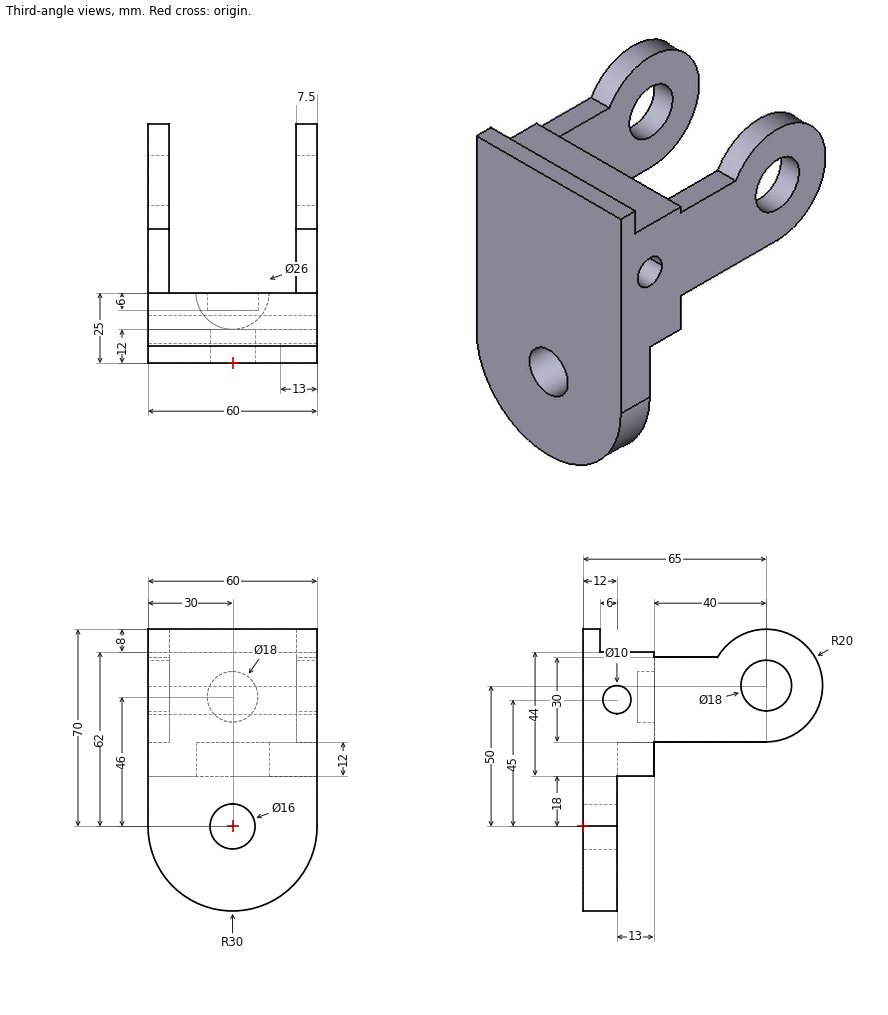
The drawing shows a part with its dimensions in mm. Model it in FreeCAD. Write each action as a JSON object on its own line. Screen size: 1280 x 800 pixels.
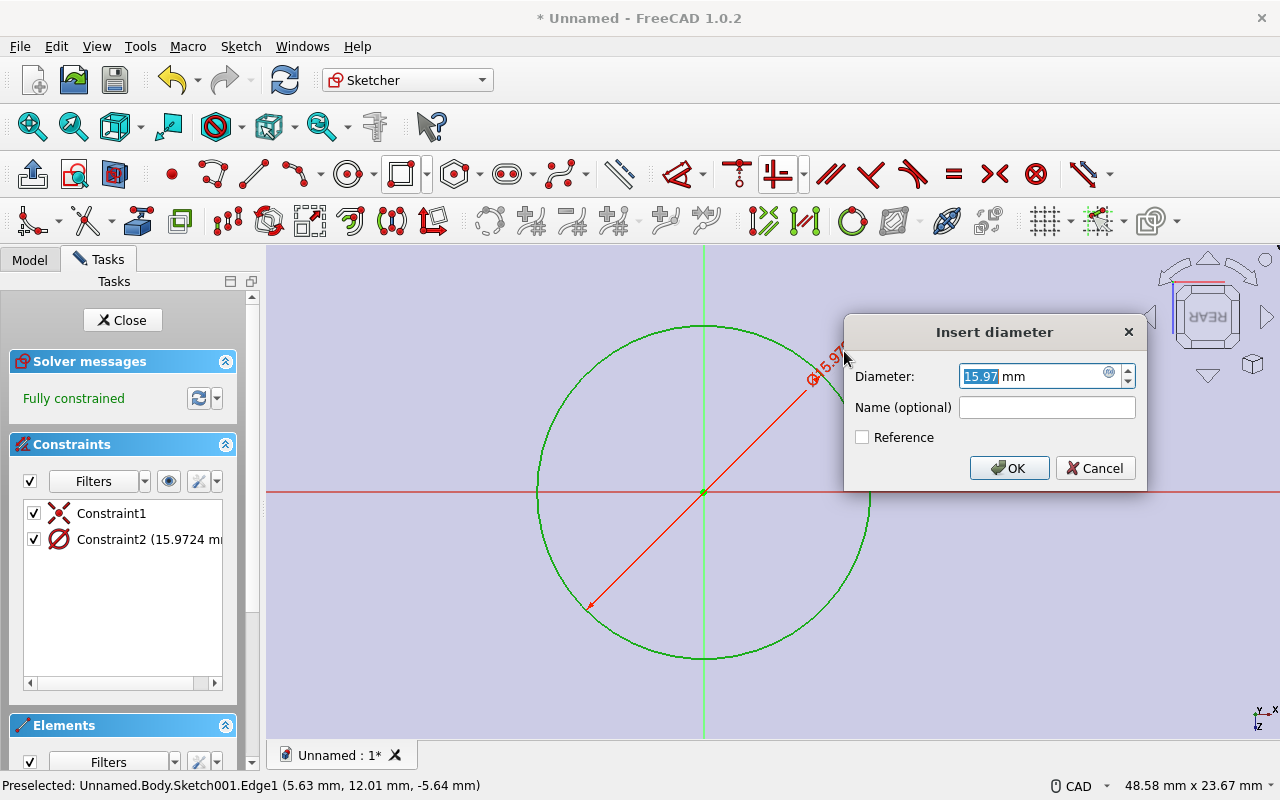
{"action": "type", "text": "16"}
{"action": "key", "text": "Return"}
{"action": "key", "text": "Escape"}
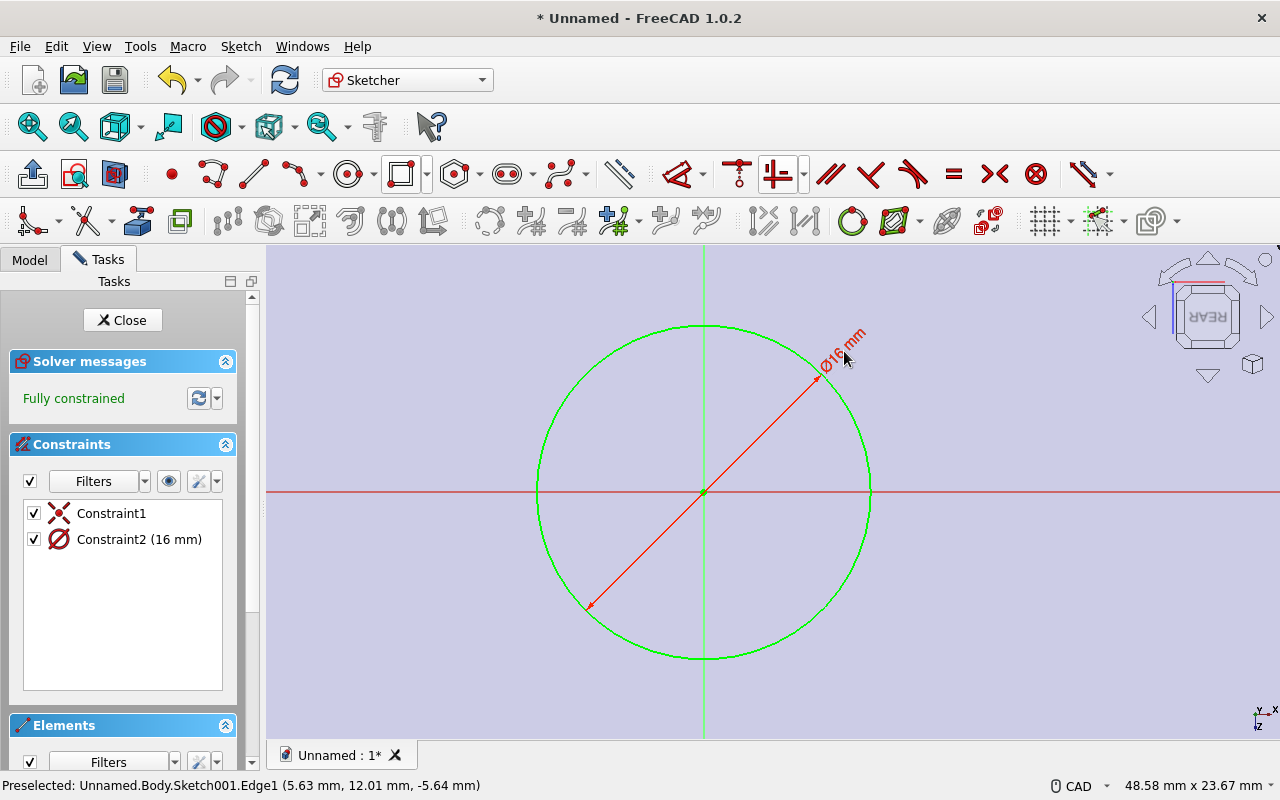
{"action": "left_click", "coordinate": [123, 320]}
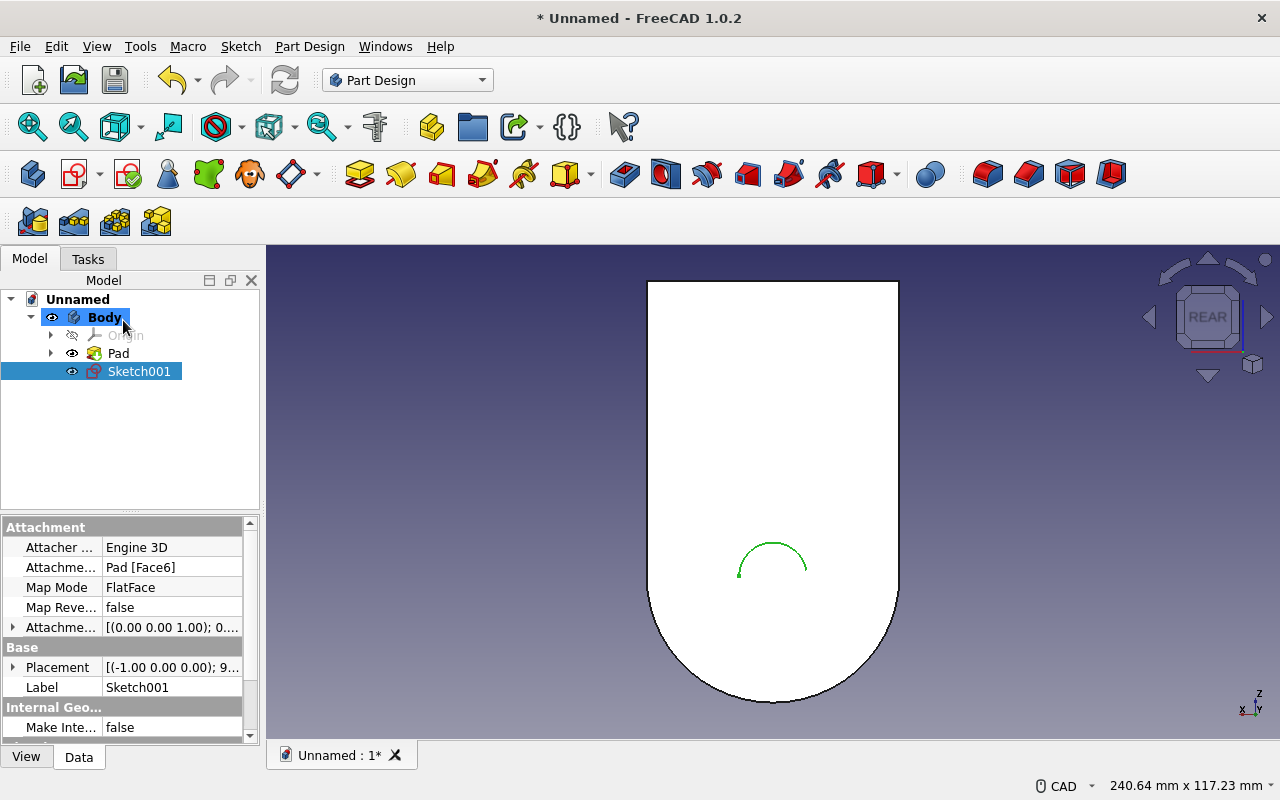
{"action": "left_click", "coordinate": [625, 174]}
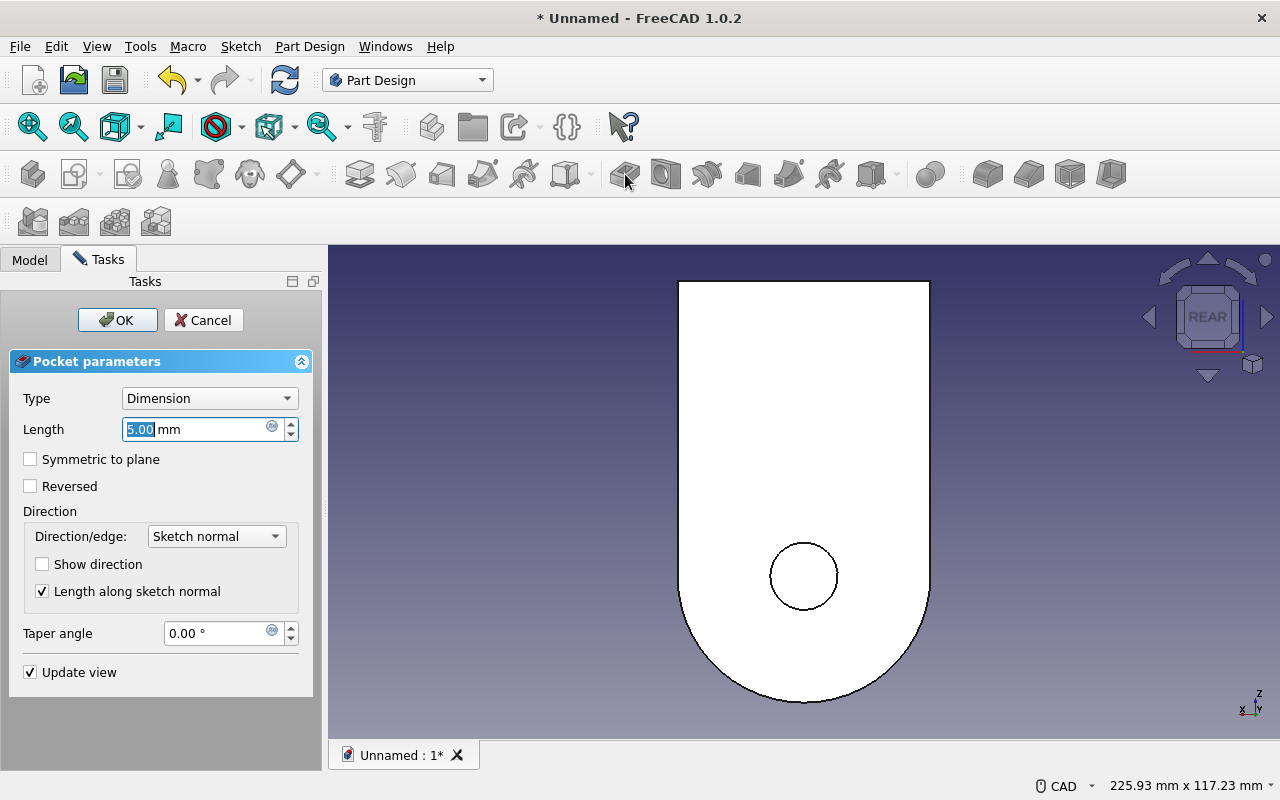
{"action": "type", "text": "12"}
{"action": "key", "text": "Tab"}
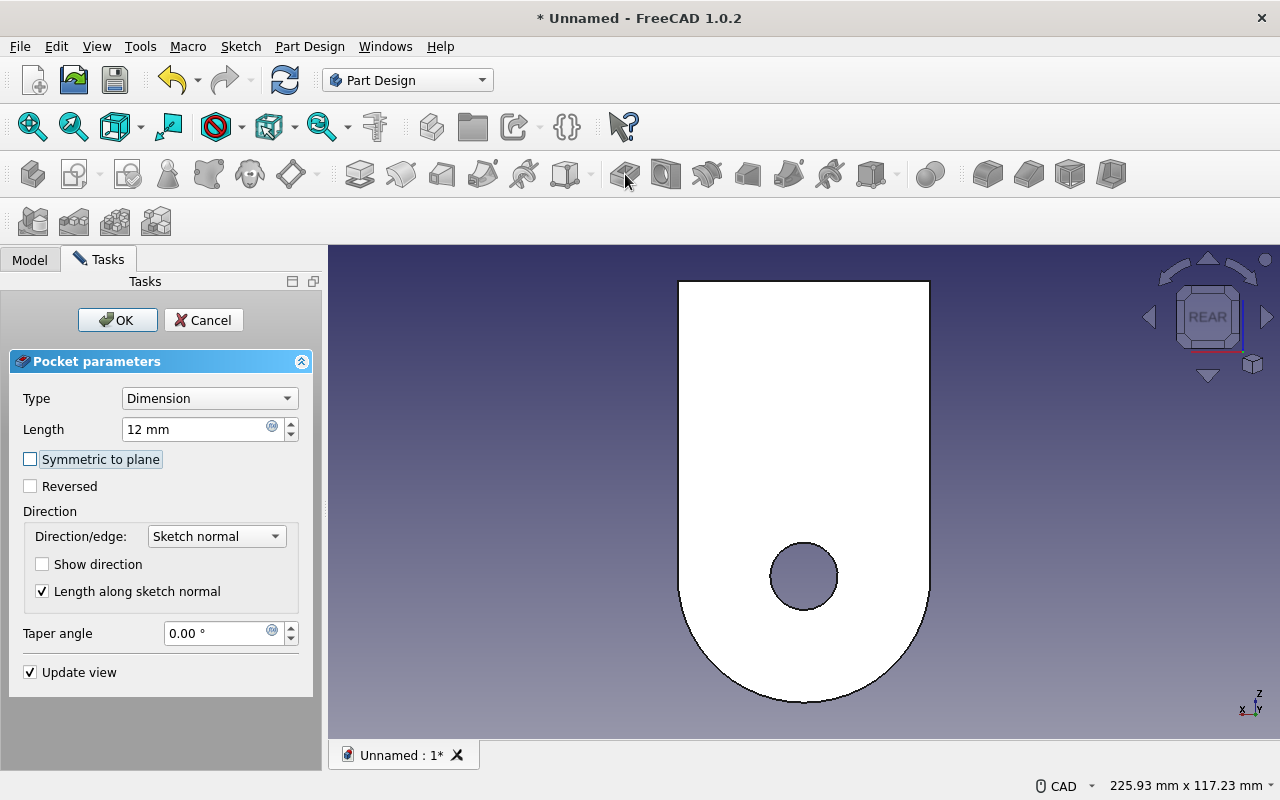
{"action": "left_click", "coordinate": [118, 320]}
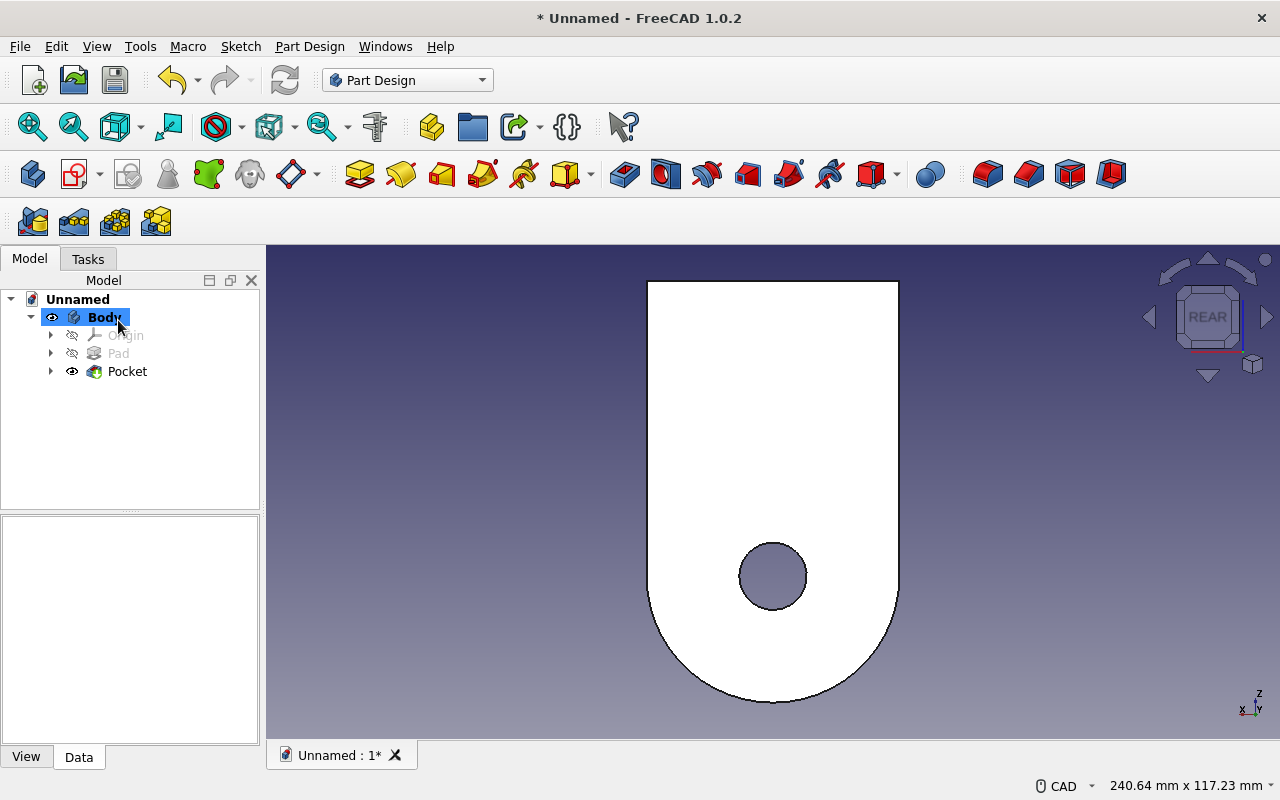
{"action": "left_click", "coordinate": [773, 431]}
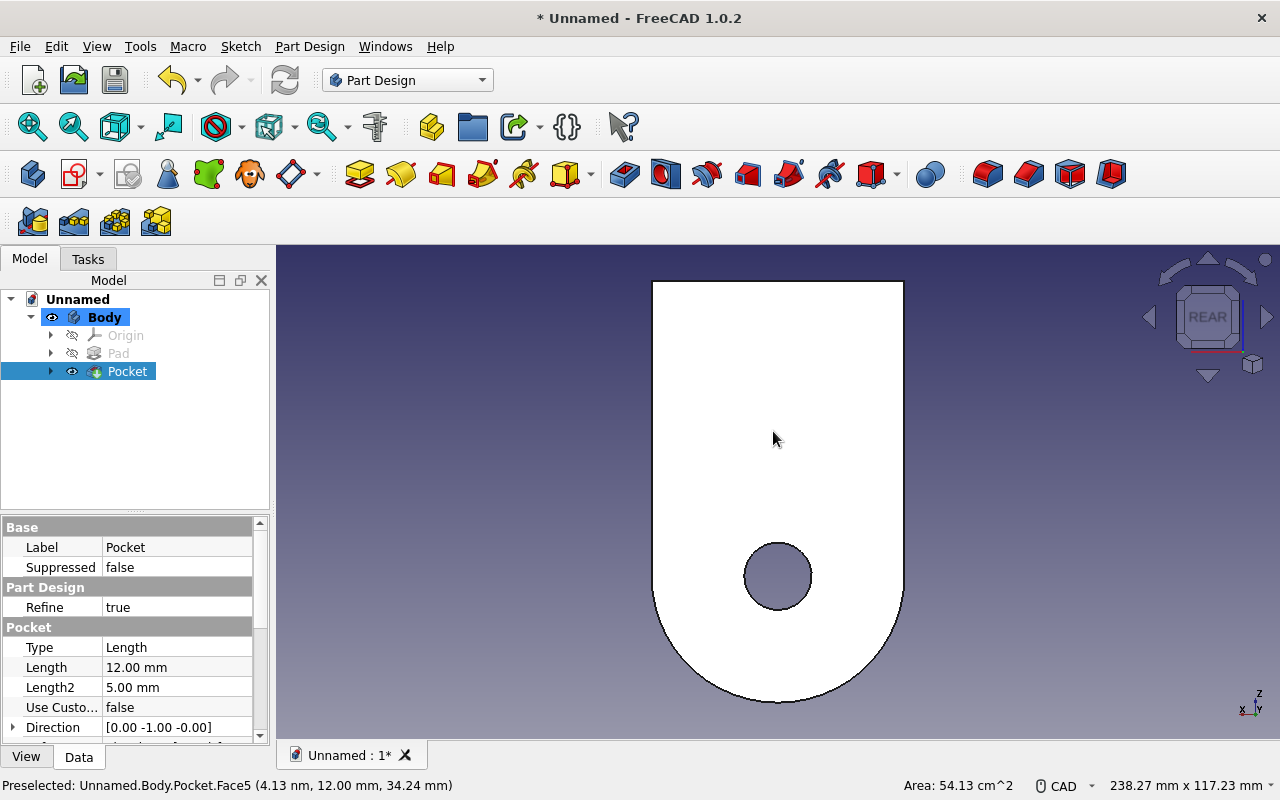
{"action": "left_click", "coordinate": [74, 174]}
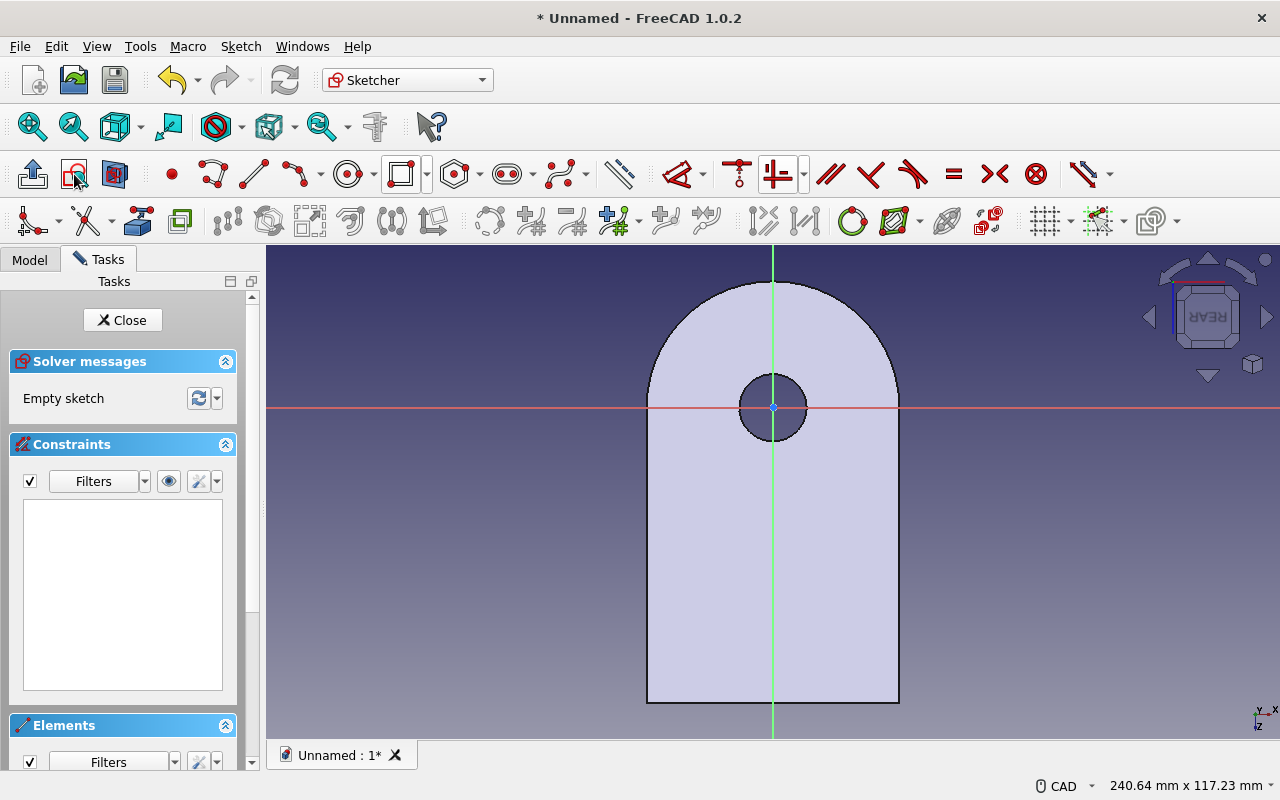
{"action": "scroll", "coordinate": [395, 273], "scroll_direction": "down", "scroll_amount": 1}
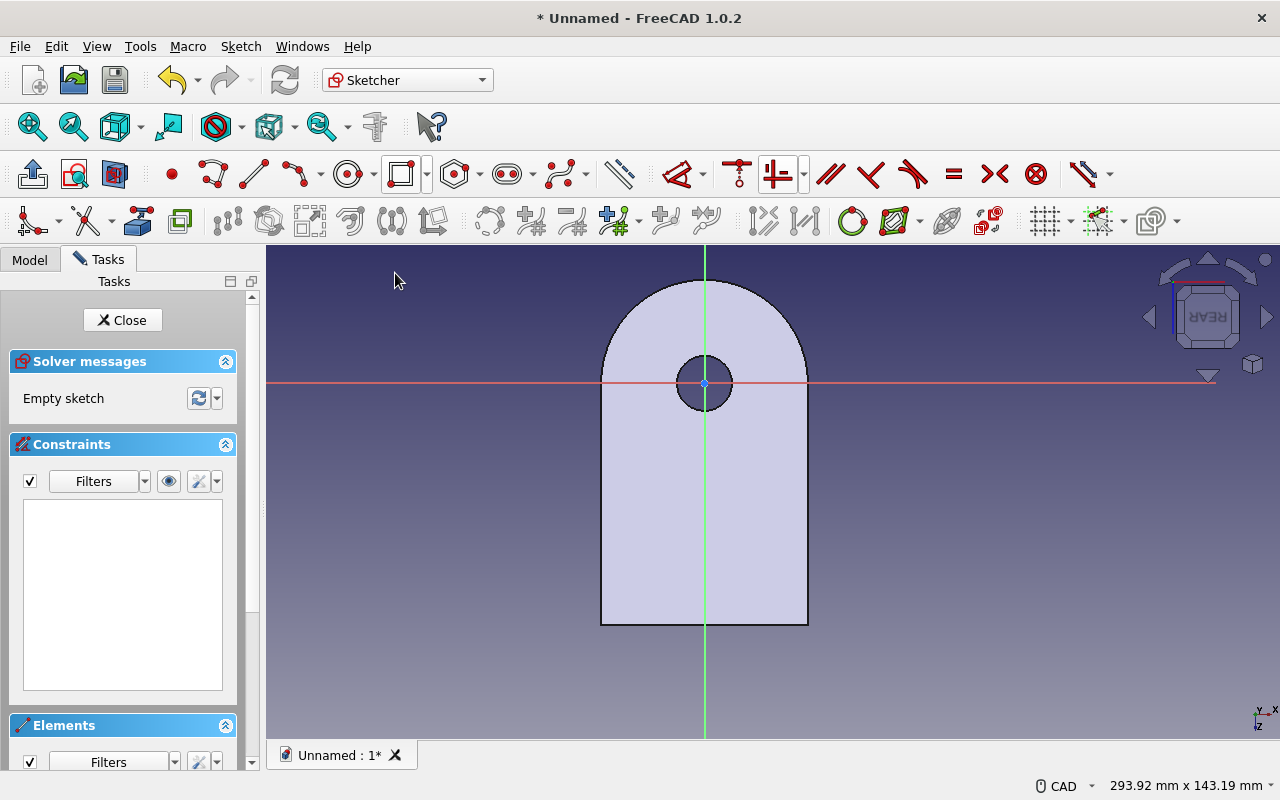
{"action": "left_click", "coordinate": [400, 174]}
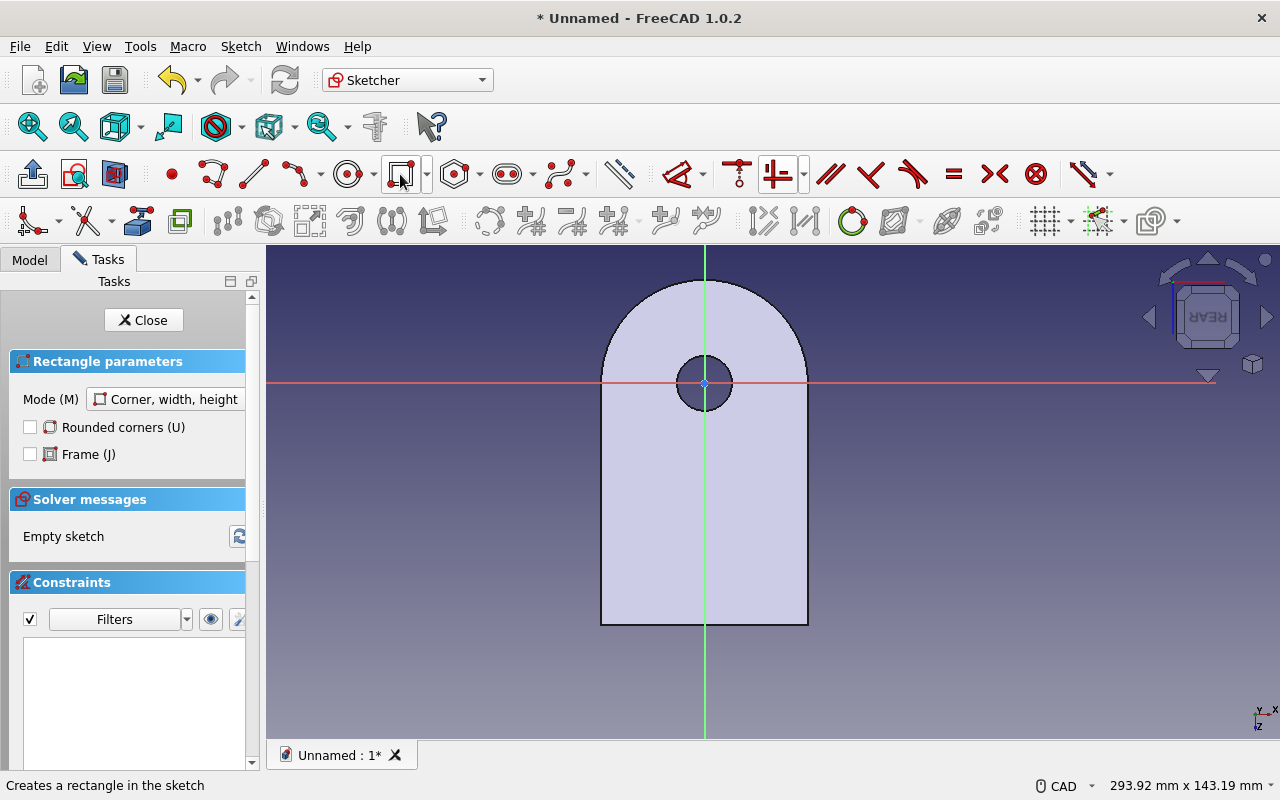
{"action": "left_click", "coordinate": [601, 597]}
{"action": "left_click", "coordinate": [808, 625]}
{"action": "key", "text": "Escape"}